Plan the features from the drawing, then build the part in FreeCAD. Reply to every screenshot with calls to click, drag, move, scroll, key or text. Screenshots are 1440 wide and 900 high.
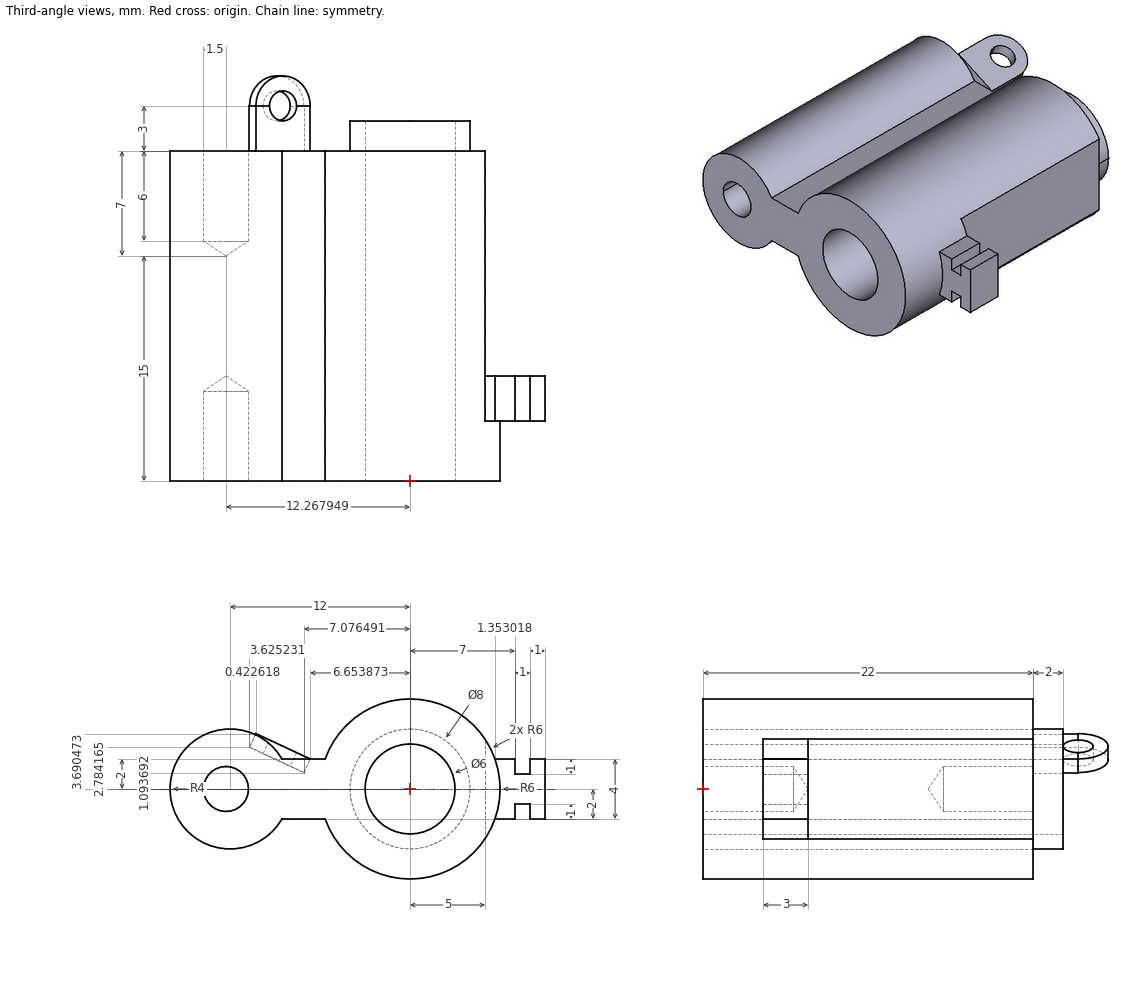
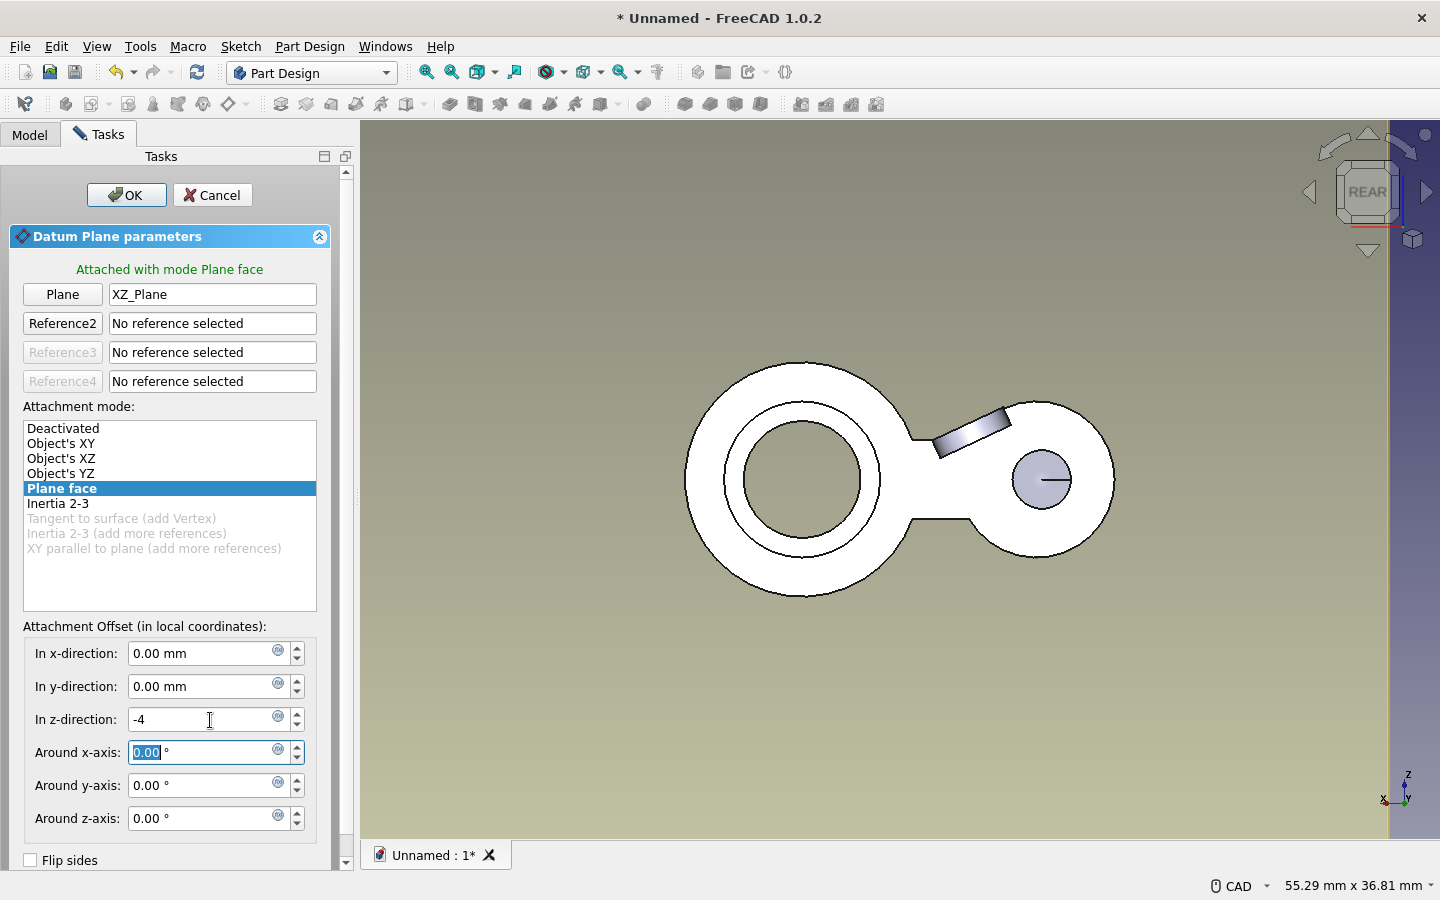
click(127, 195)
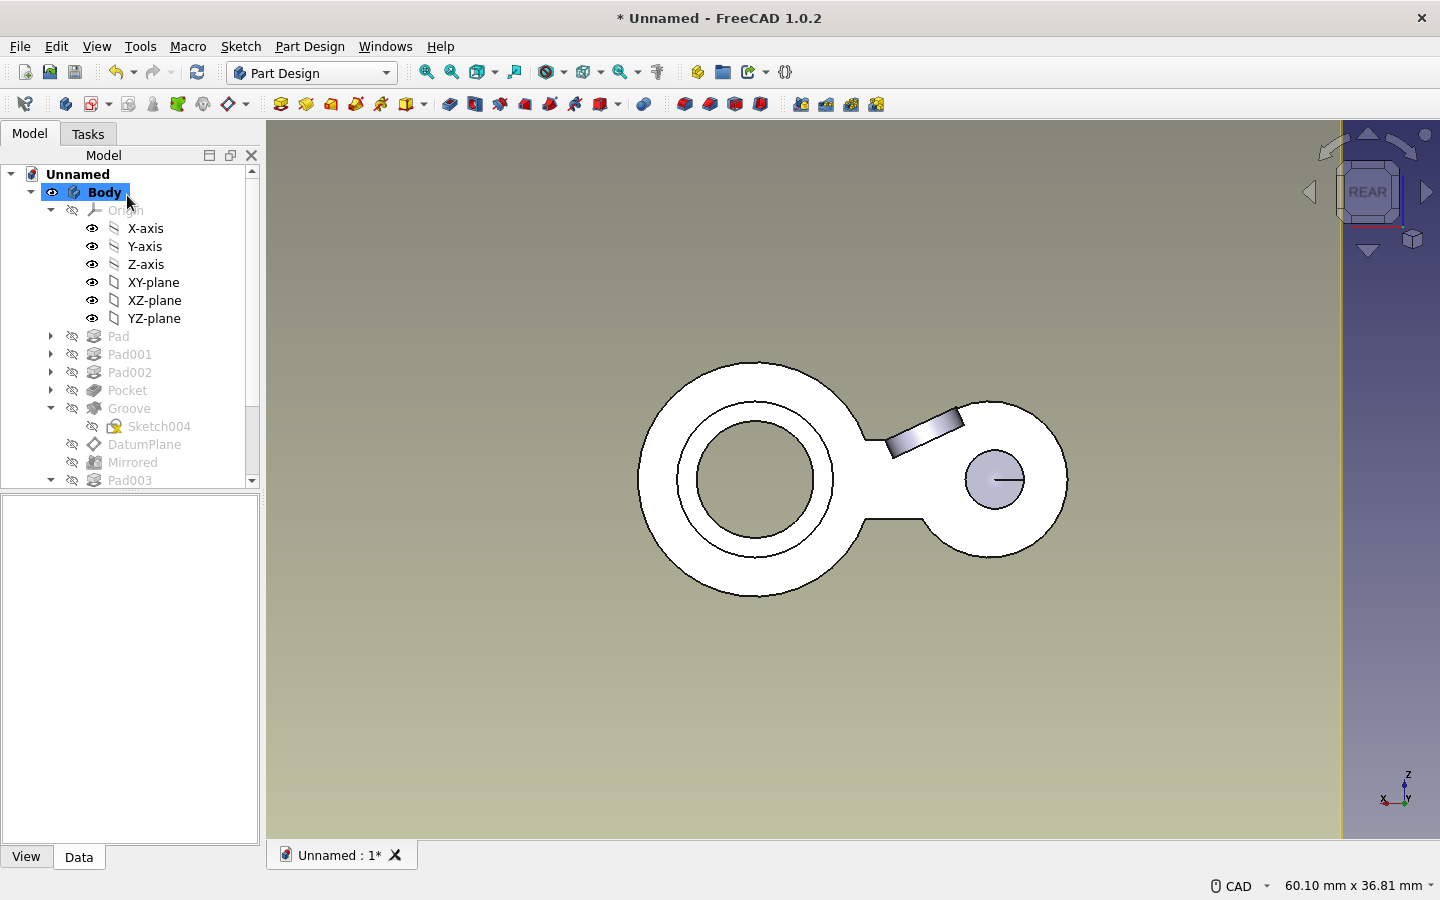
scroll(101, 332, down, 3)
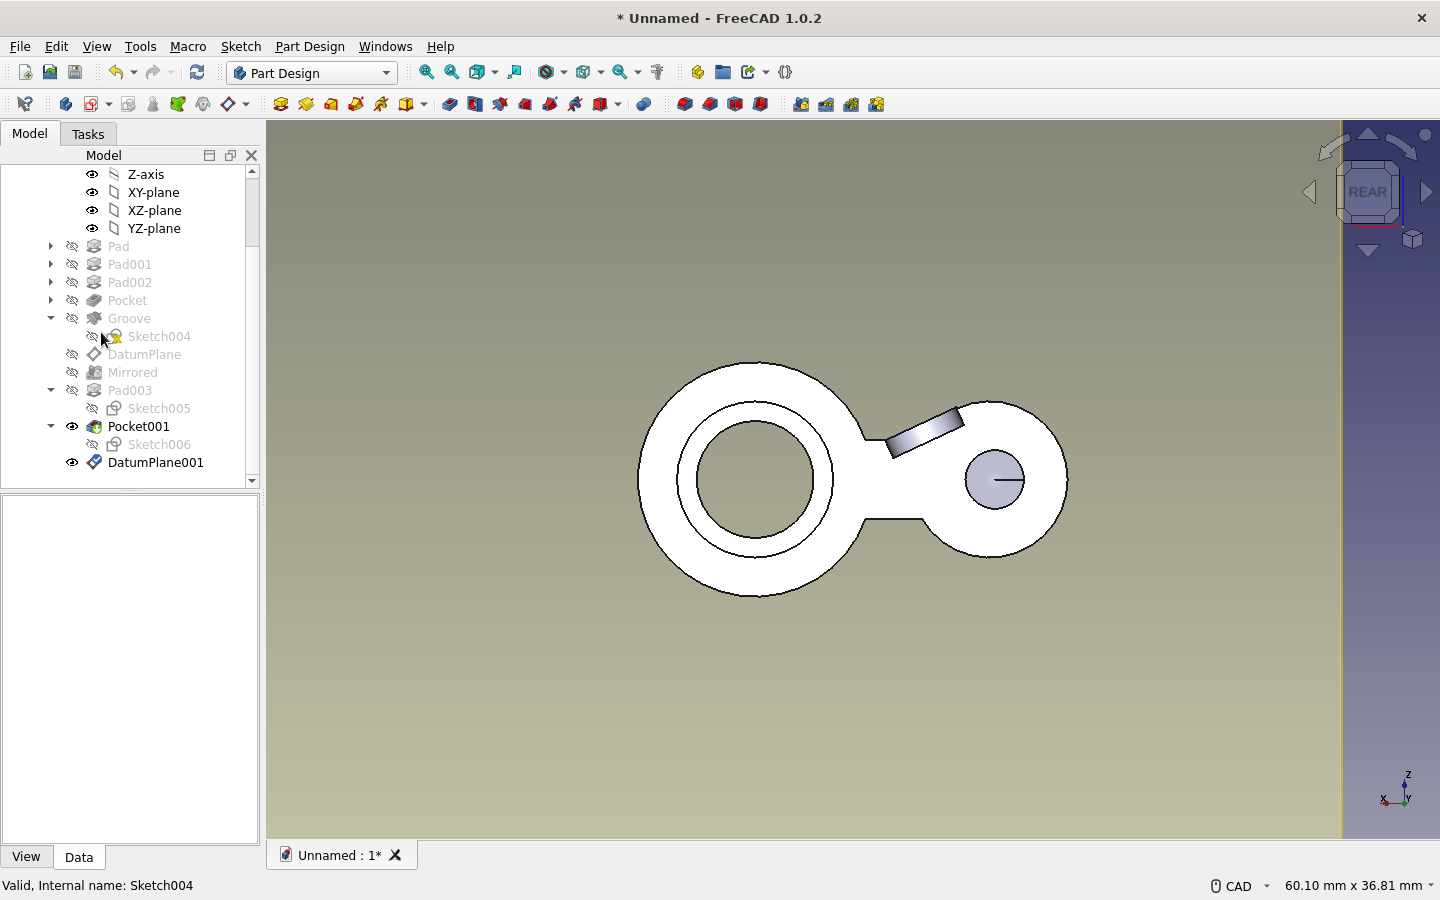
click(117, 462)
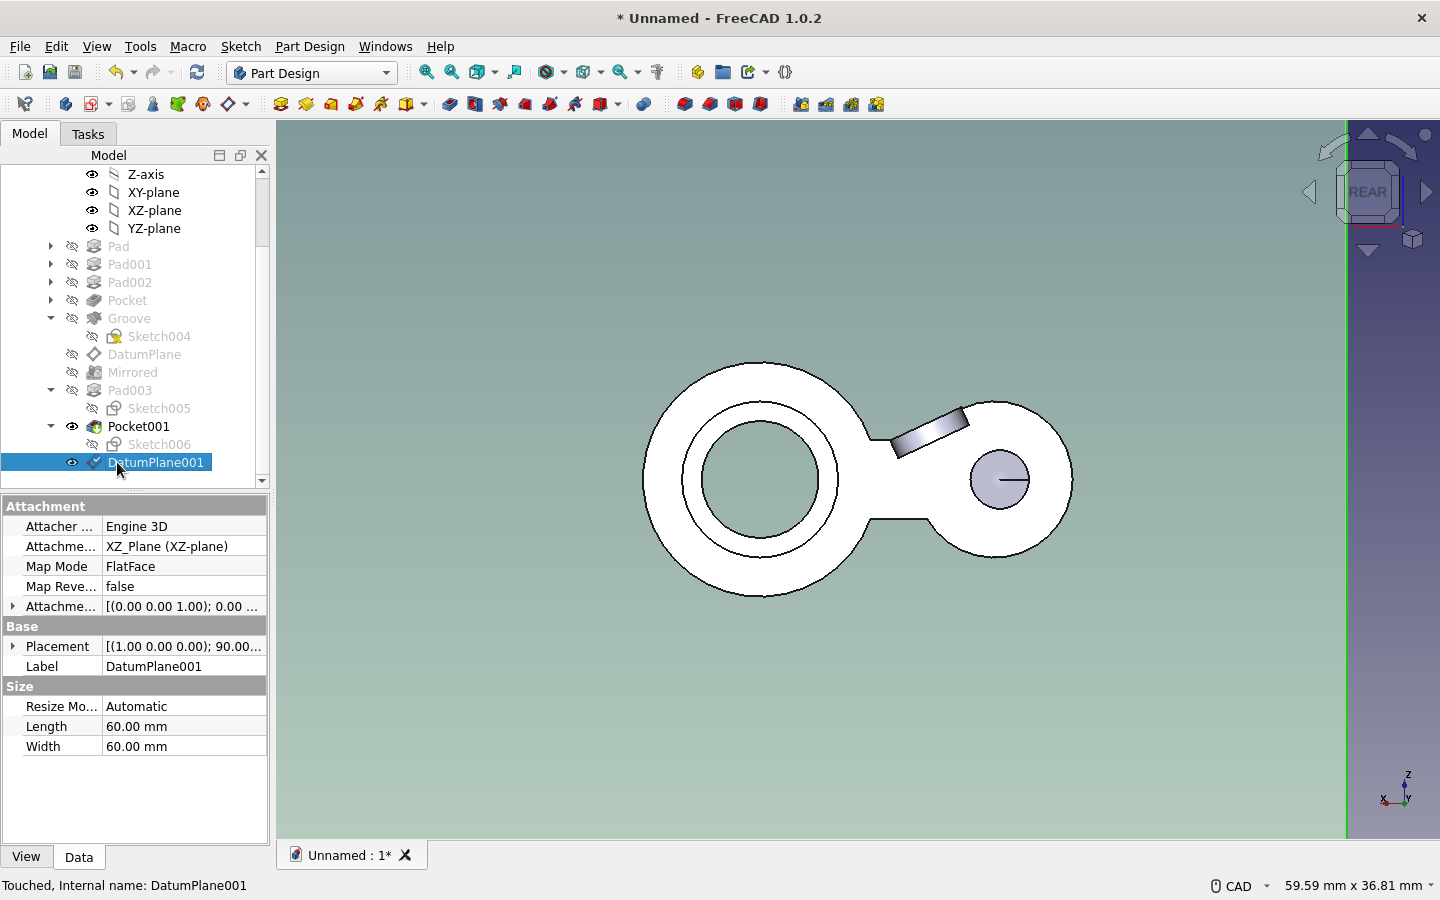
click(90, 104)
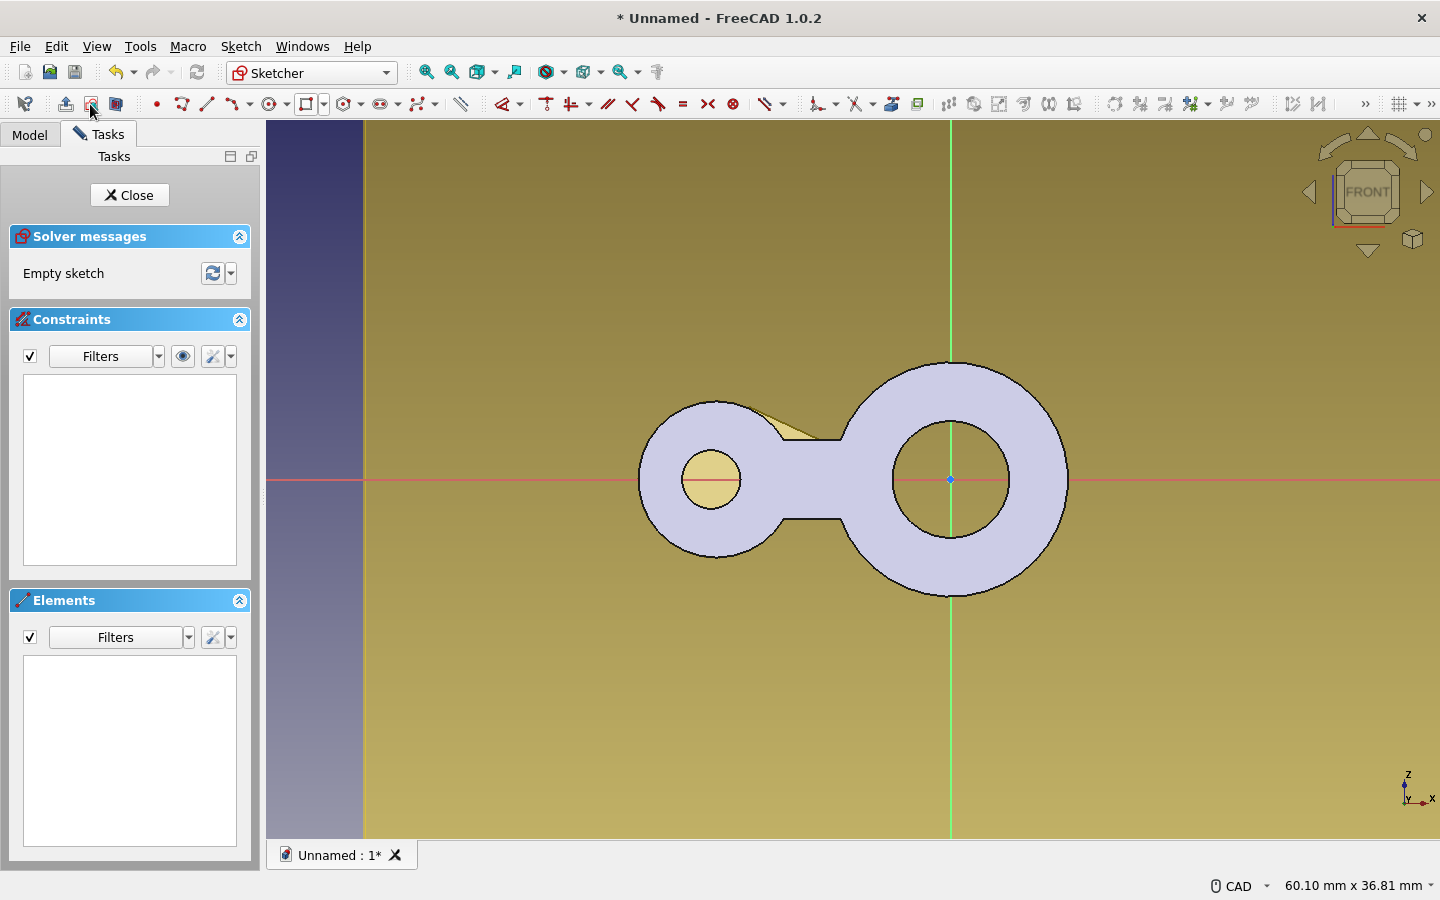
click(116, 104)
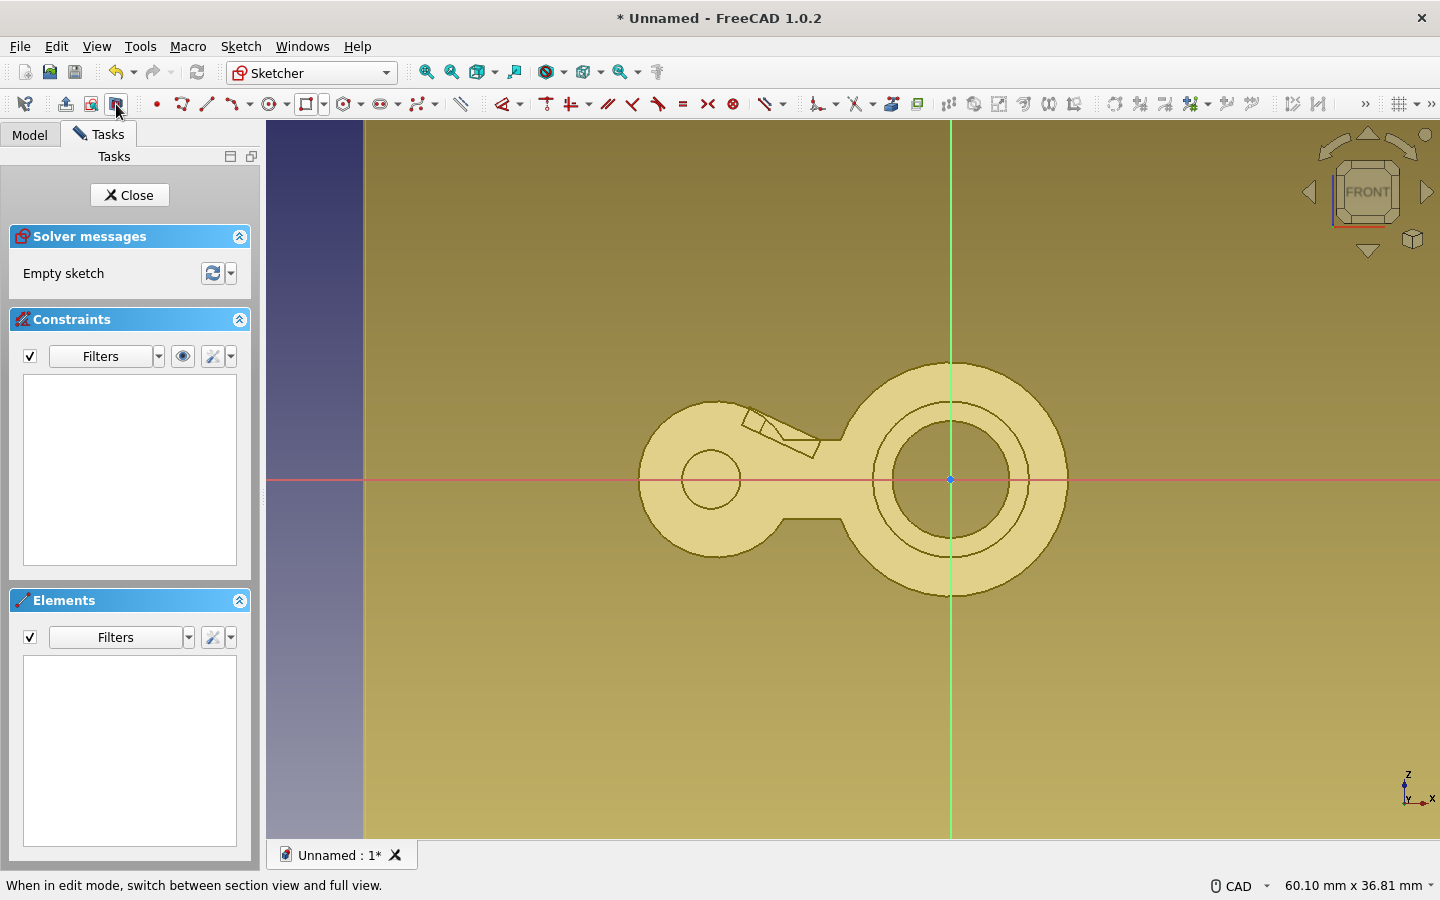
scroll(1148, 480, up, 6)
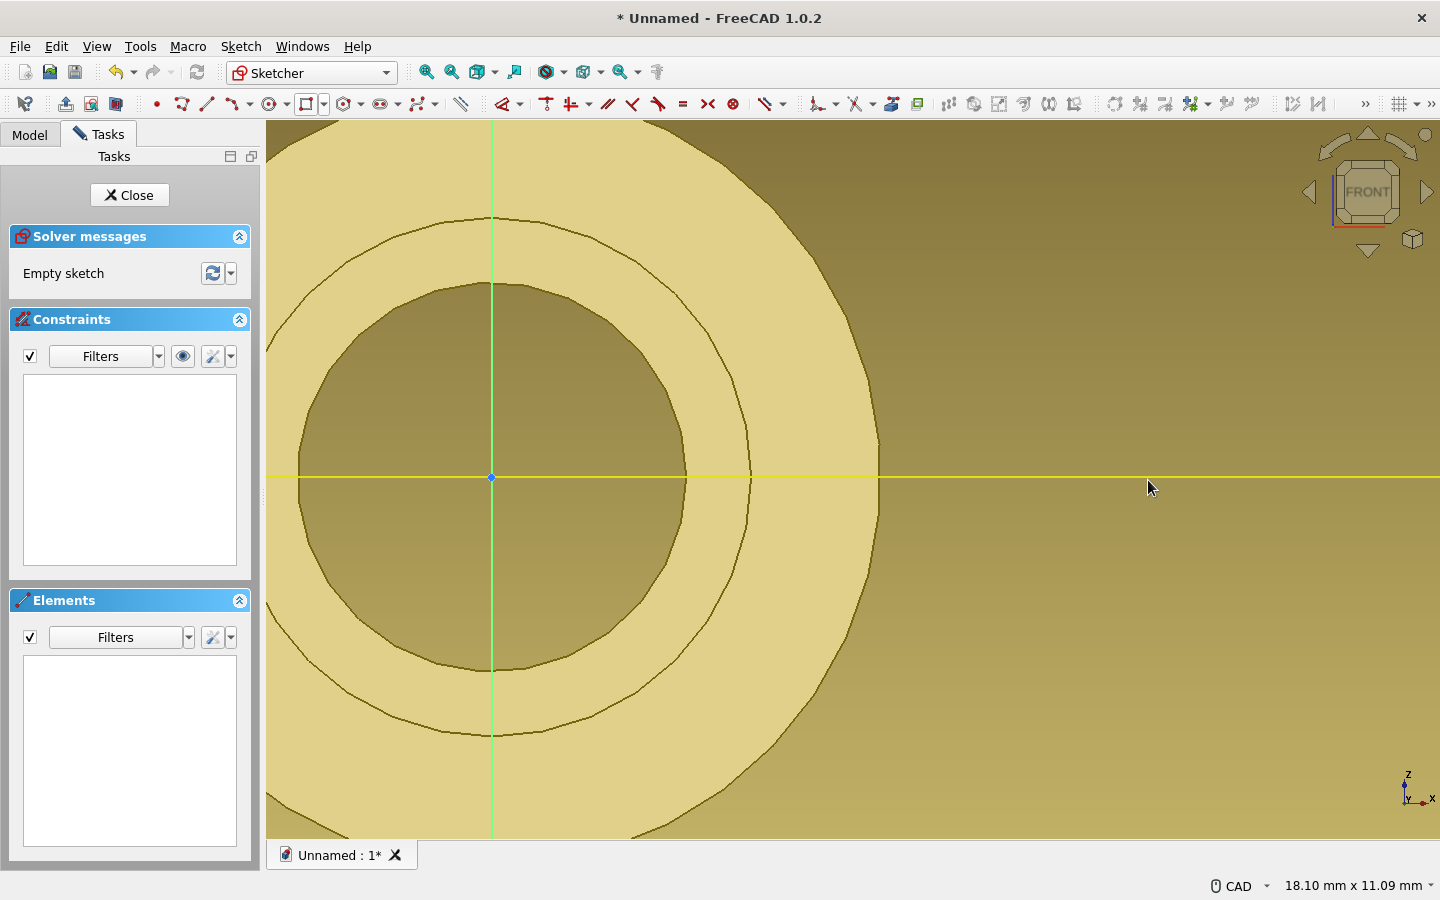
click(207, 104)